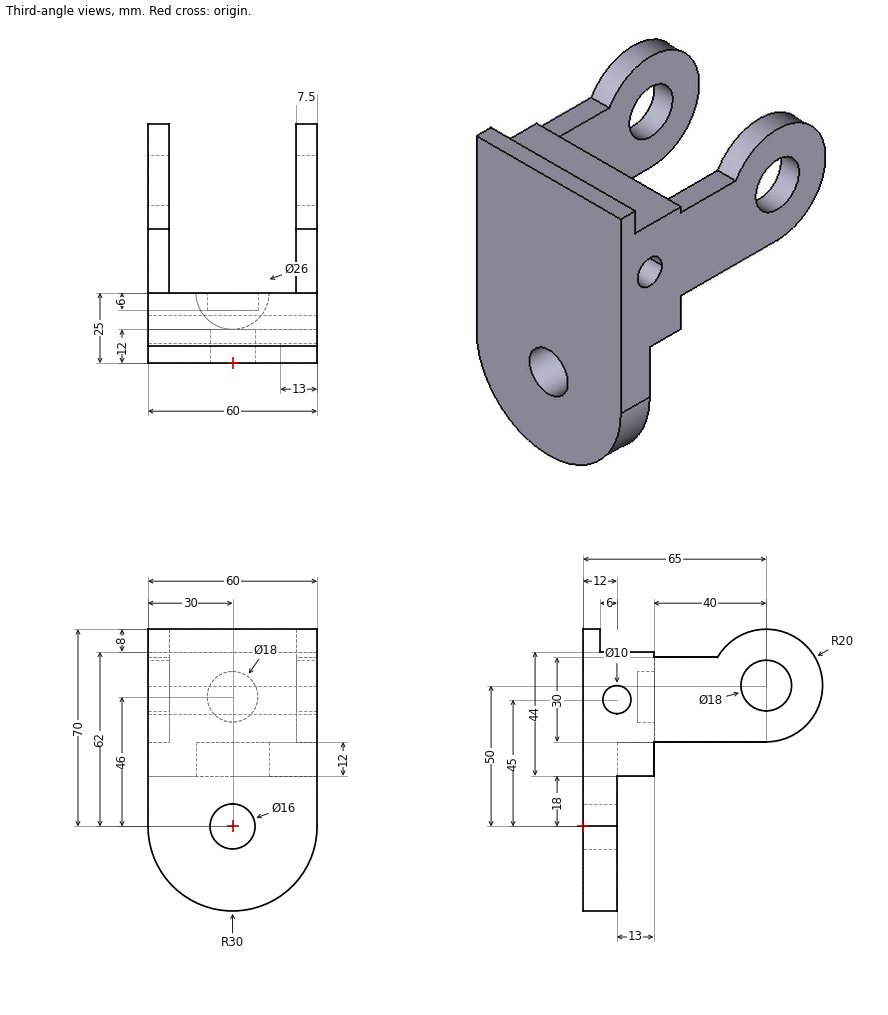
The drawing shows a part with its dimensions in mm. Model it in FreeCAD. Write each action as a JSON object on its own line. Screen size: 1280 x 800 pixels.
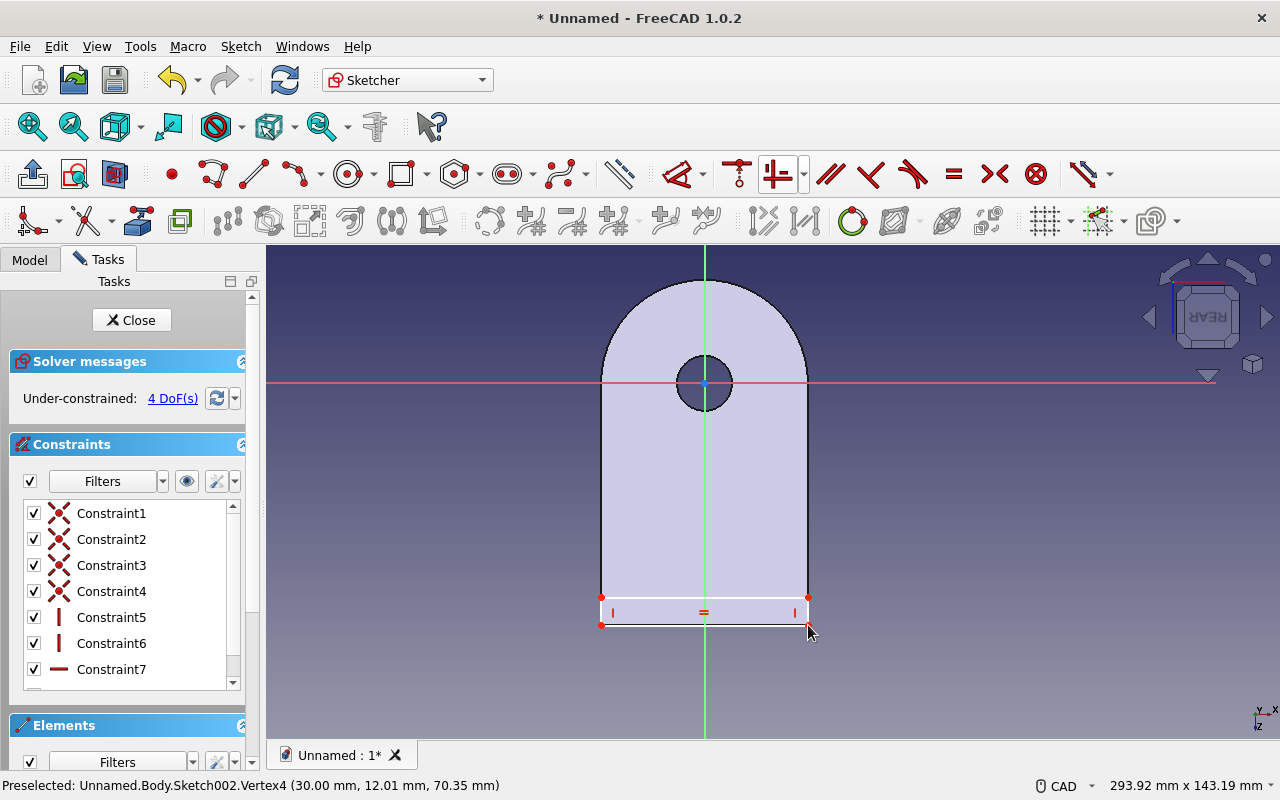
{"action": "key", "text": "d"}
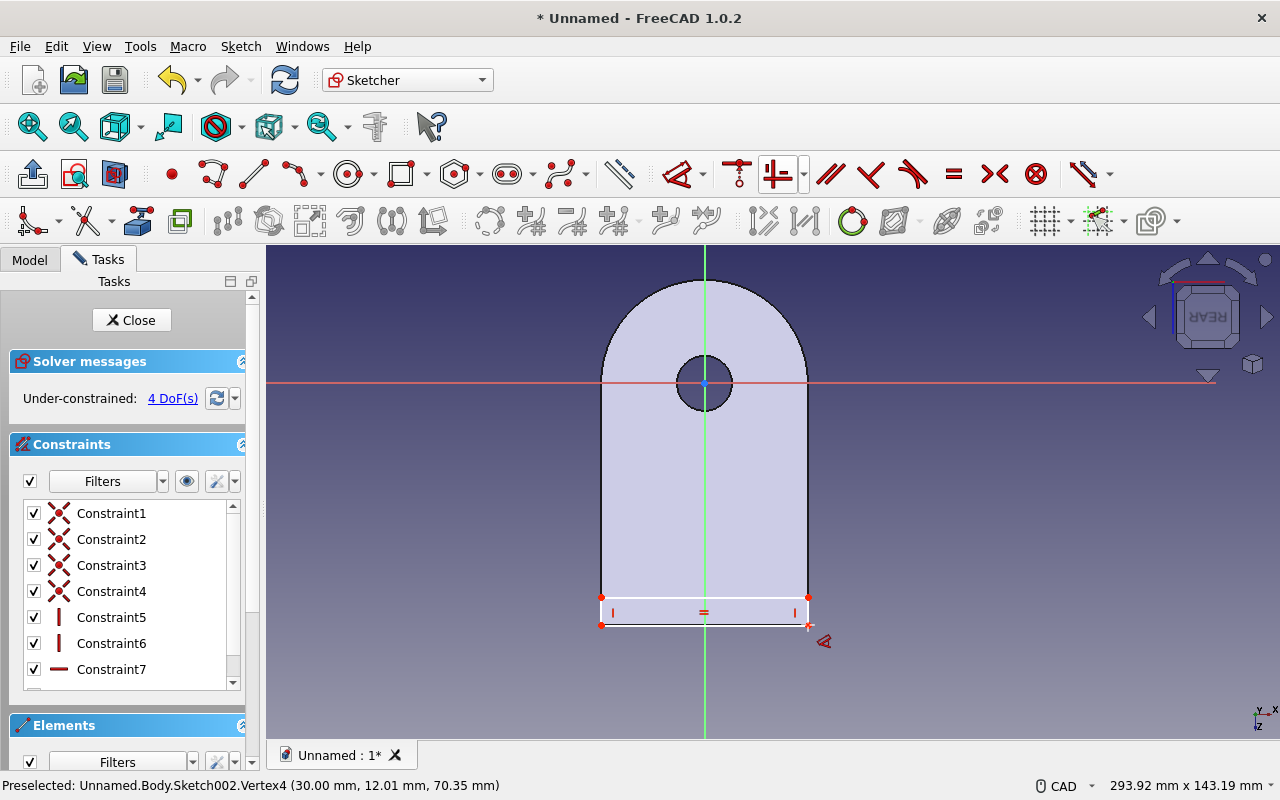
{"action": "scroll", "coordinate": [601, 609], "scroll_direction": "up", "scroll_amount": 2}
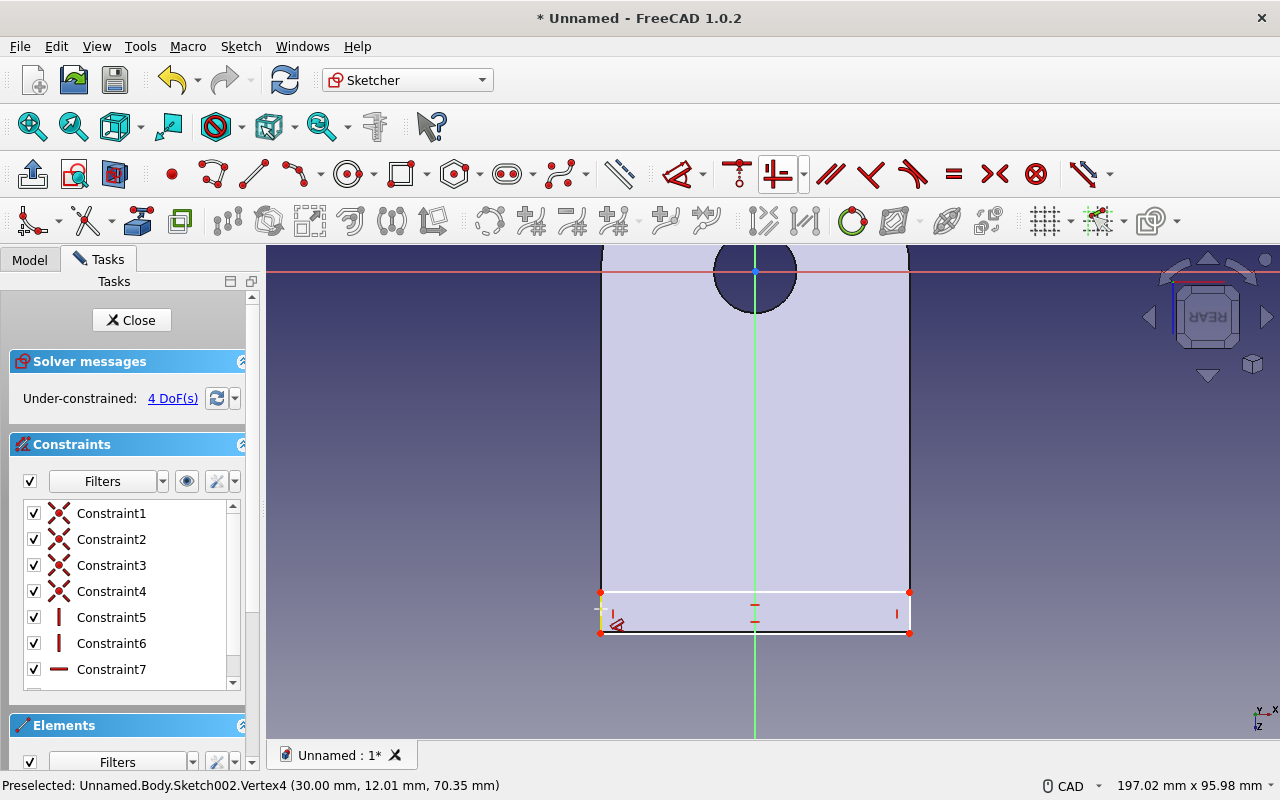
{"action": "left_click", "coordinate": [601, 609]}
{"action": "left_click", "coordinate": [567, 613]}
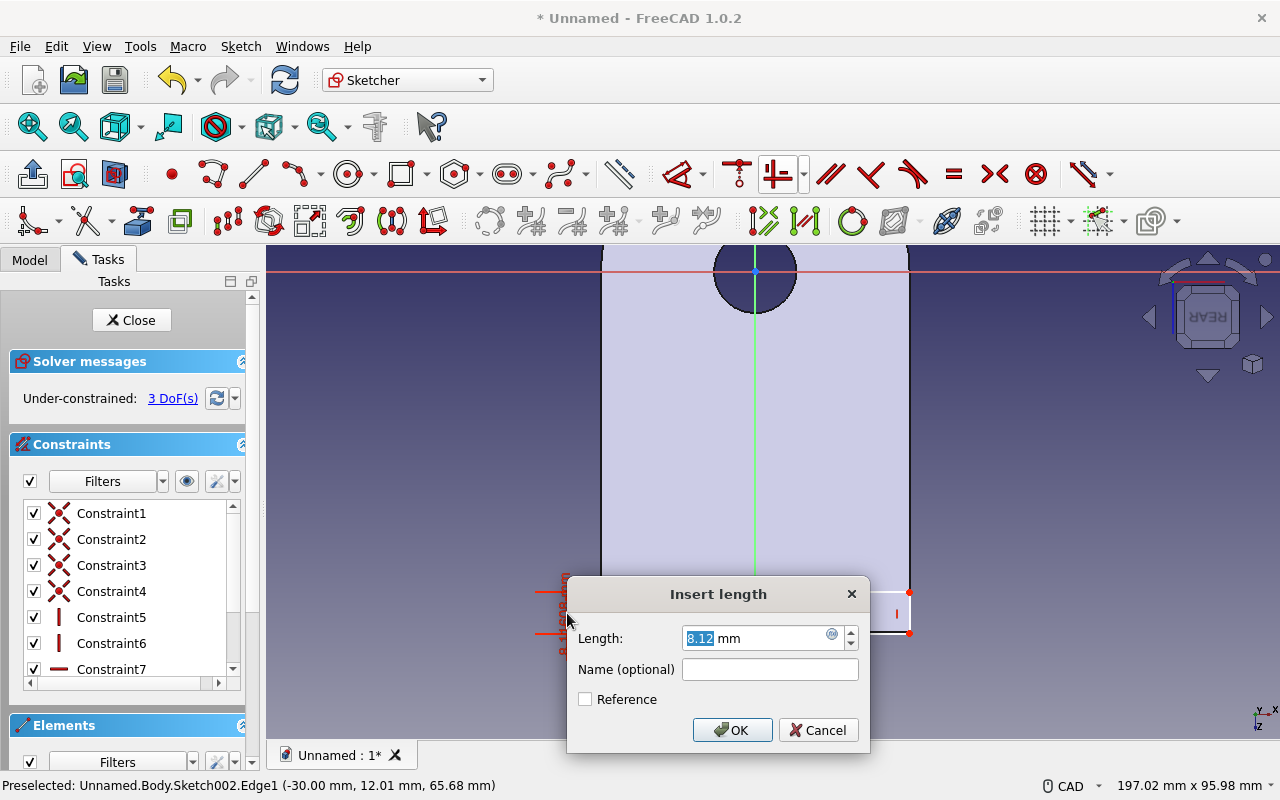
{"action": "type", "text": "8"}
{"action": "key", "text": "Return"}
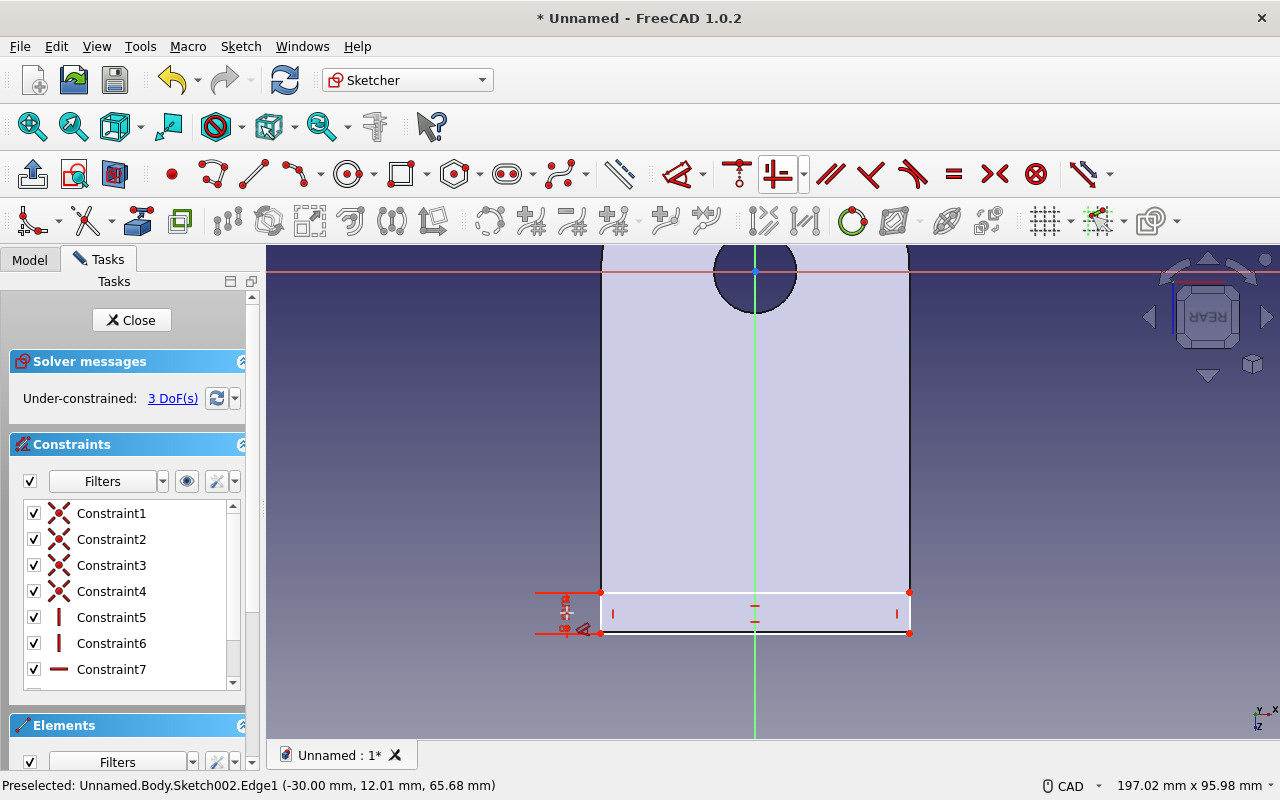
{"action": "left_click", "coordinate": [693, 634]}
{"action": "left_click", "coordinate": [684, 668]}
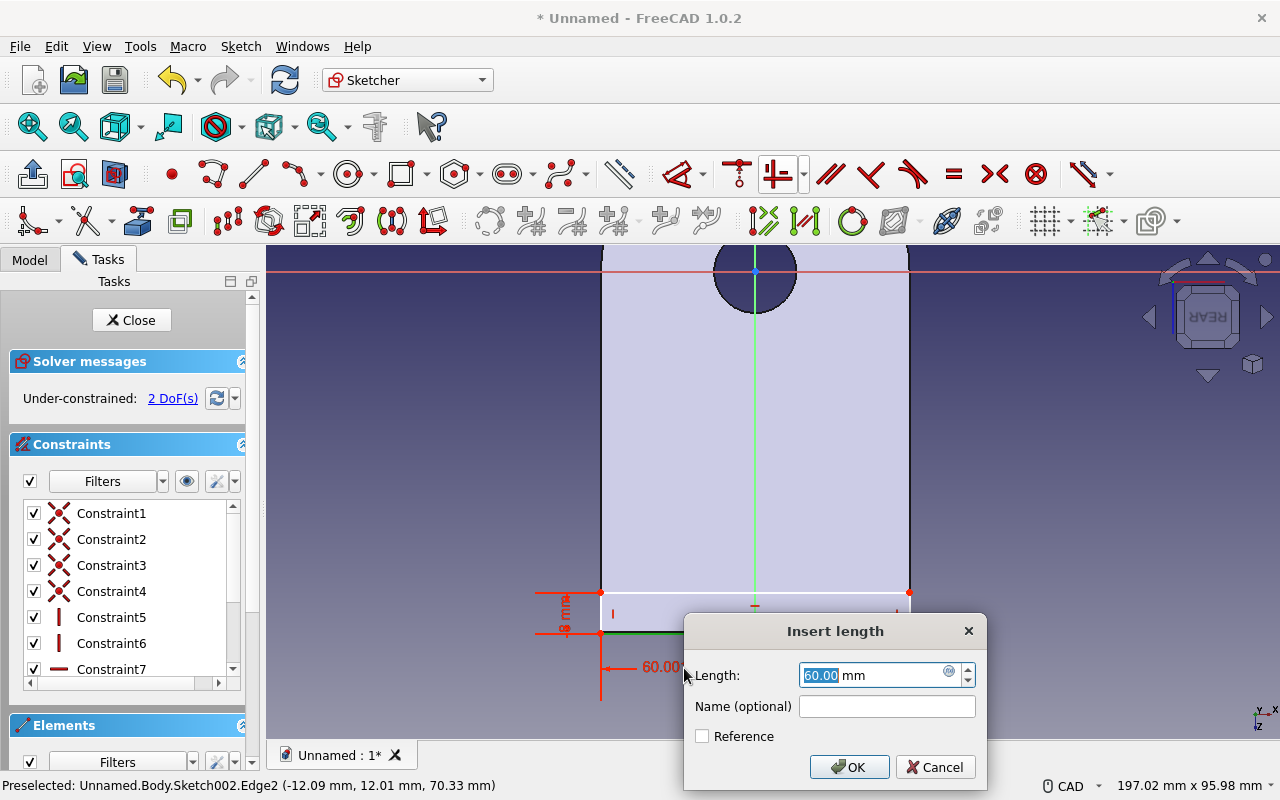
{"action": "type", "text": "60"}
{"action": "key", "text": "Return"}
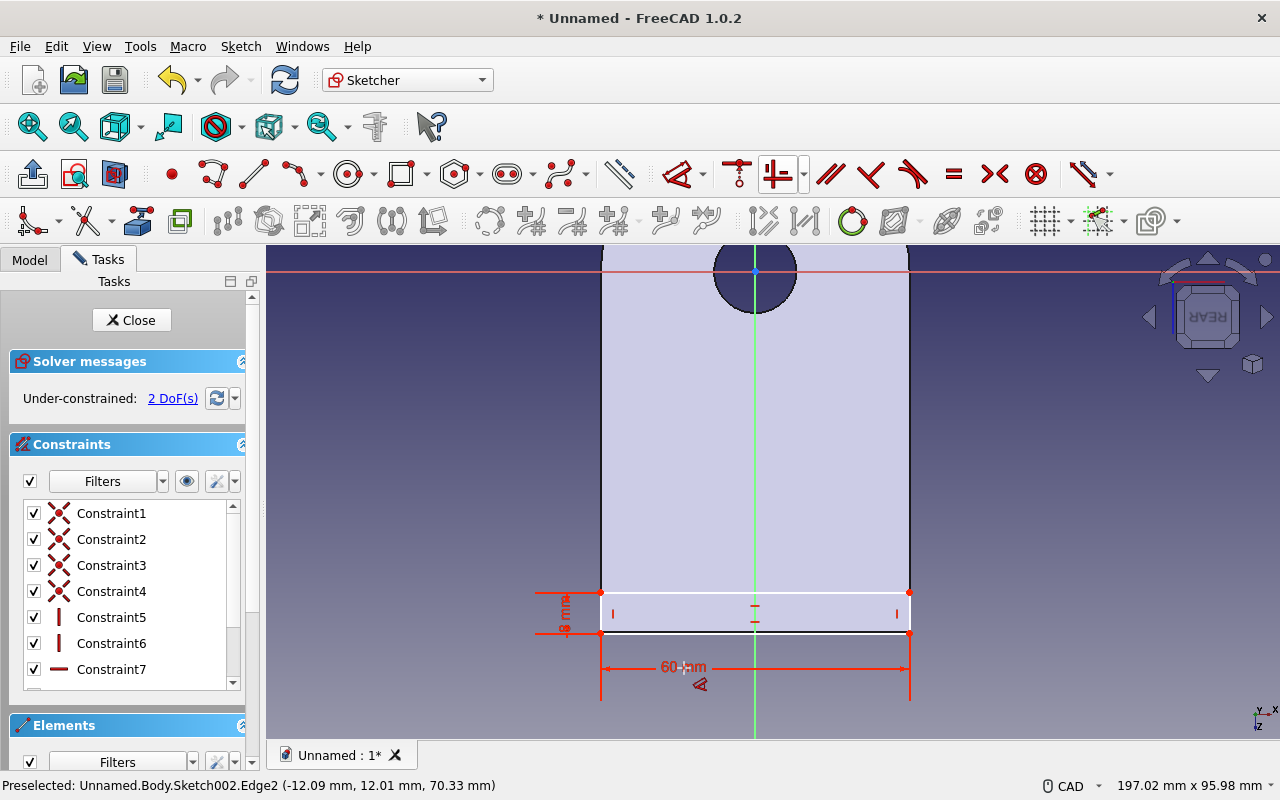
{"action": "left_click", "coordinate": [601, 593]}
{"action": "left_click", "coordinate": [678, 699]}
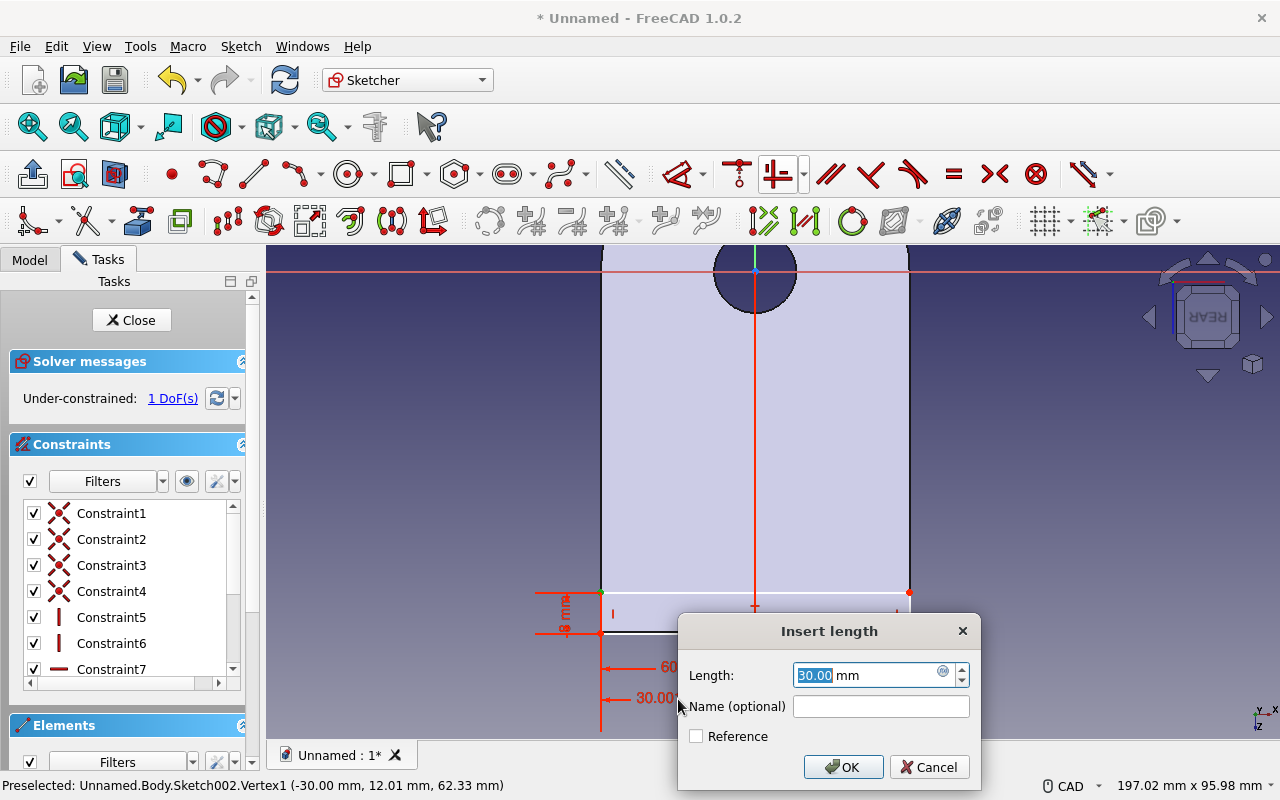
{"action": "type", "text": "30"}
{"action": "key", "text": "Return"}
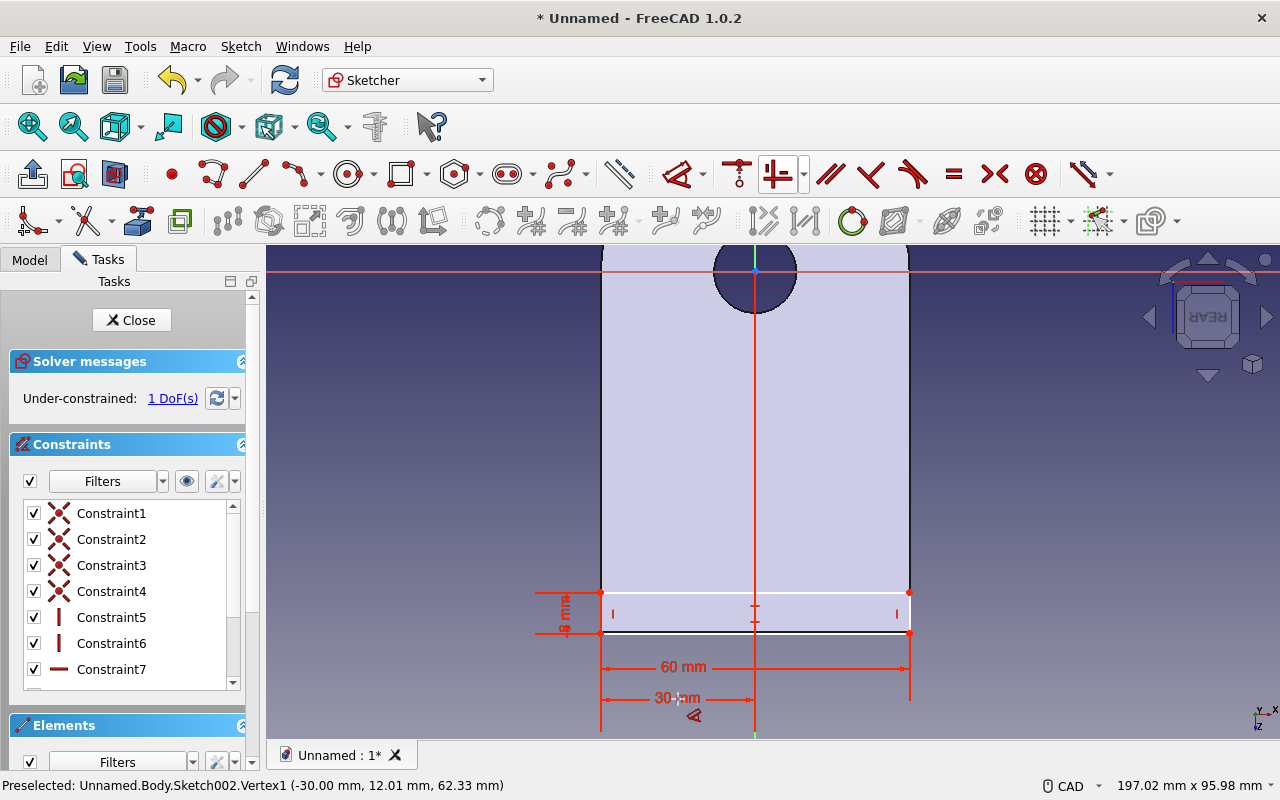
{"action": "left_click", "coordinate": [601, 593]}
{"action": "left_click", "coordinate": [567, 433]}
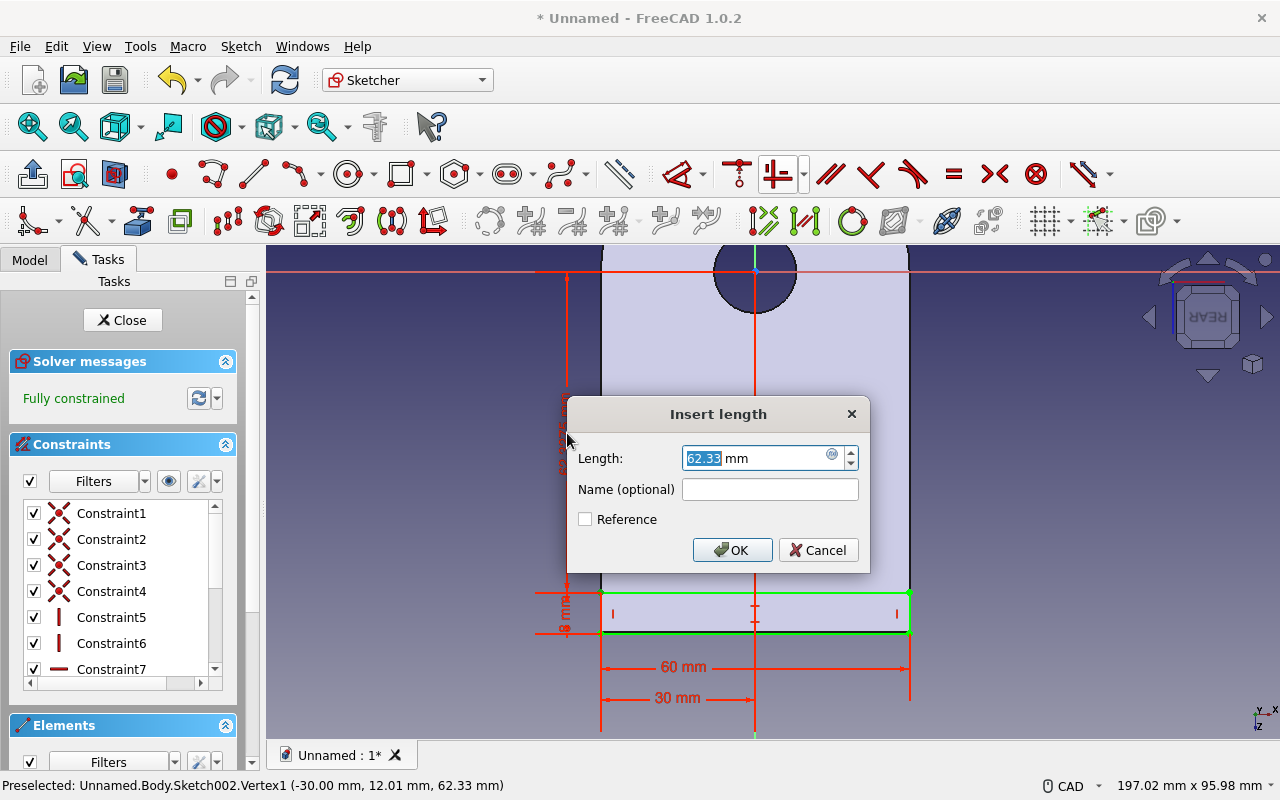
{"action": "type", "text": "62"}
{"action": "key", "text": "Return"}
{"action": "key", "text": "Escape"}